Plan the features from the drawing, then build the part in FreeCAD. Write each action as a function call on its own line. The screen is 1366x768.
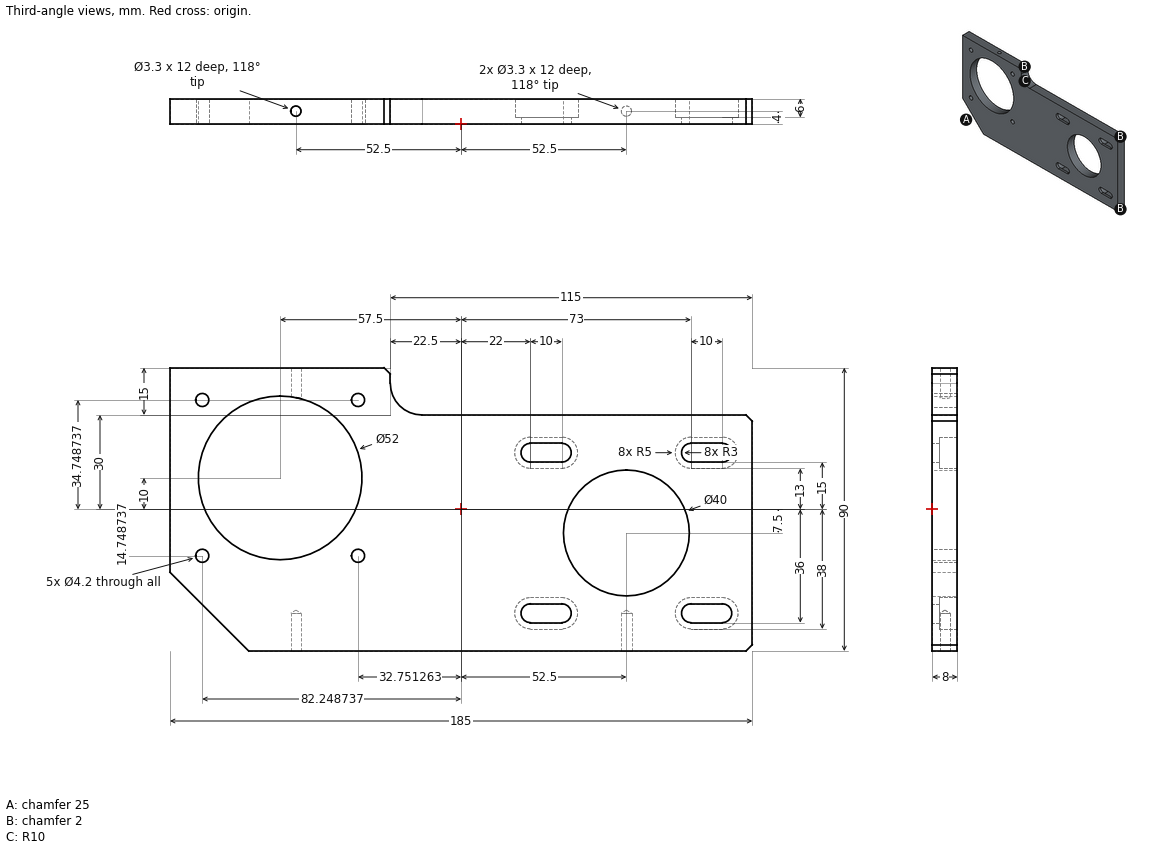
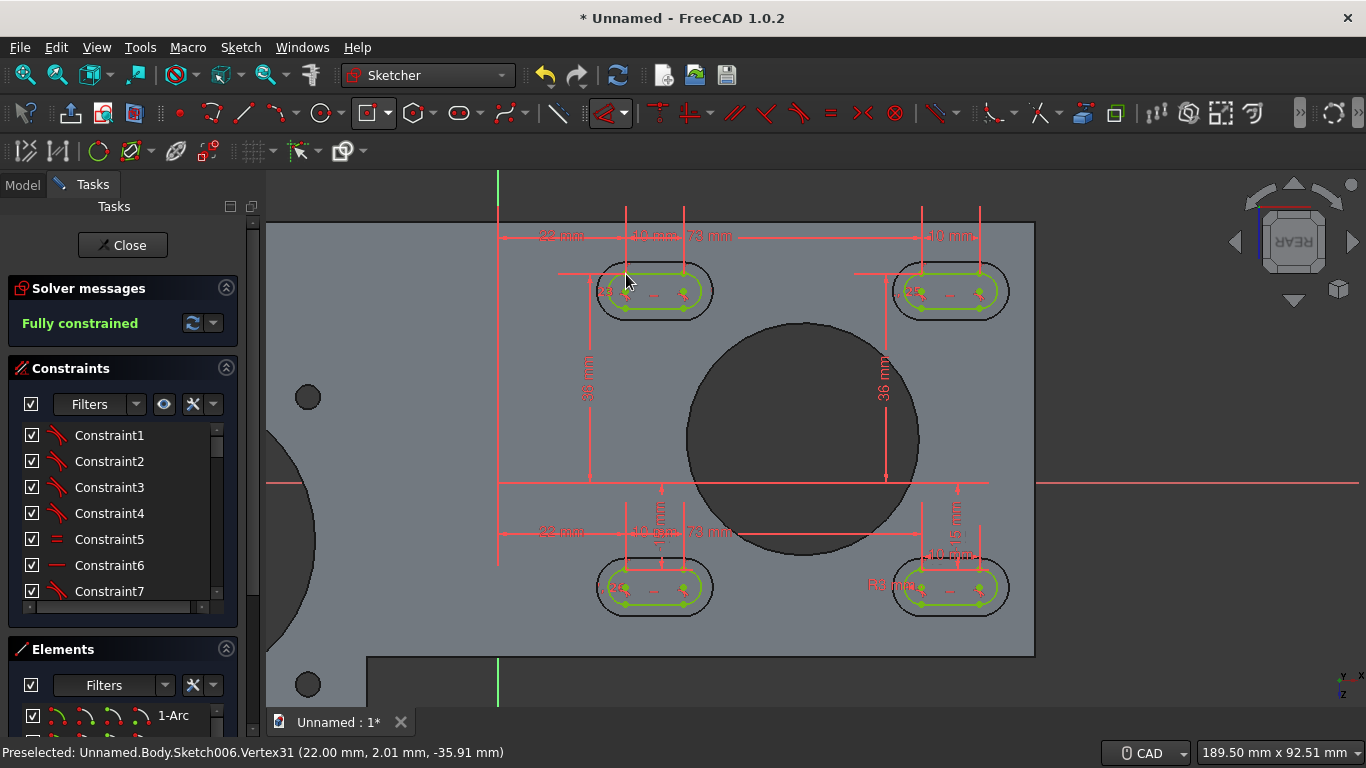
click(123, 245)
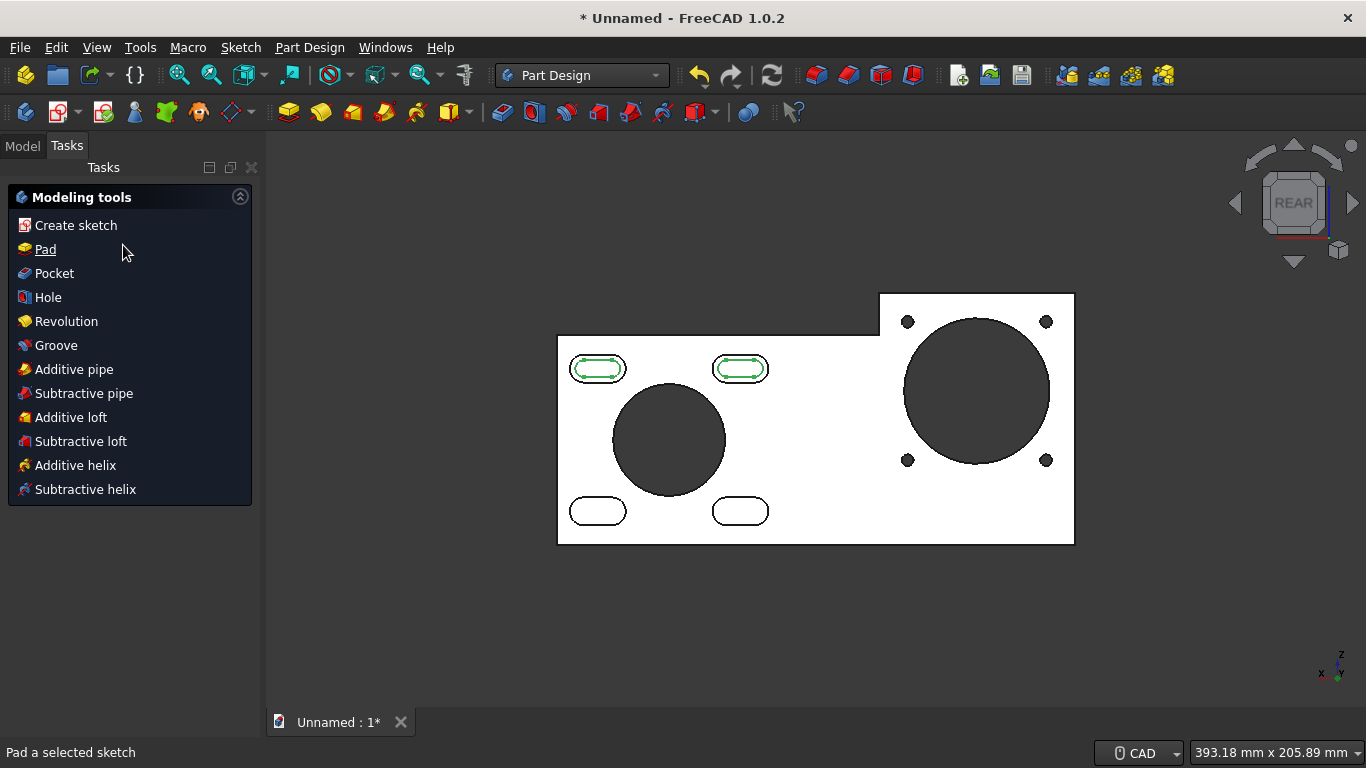
click(504, 112)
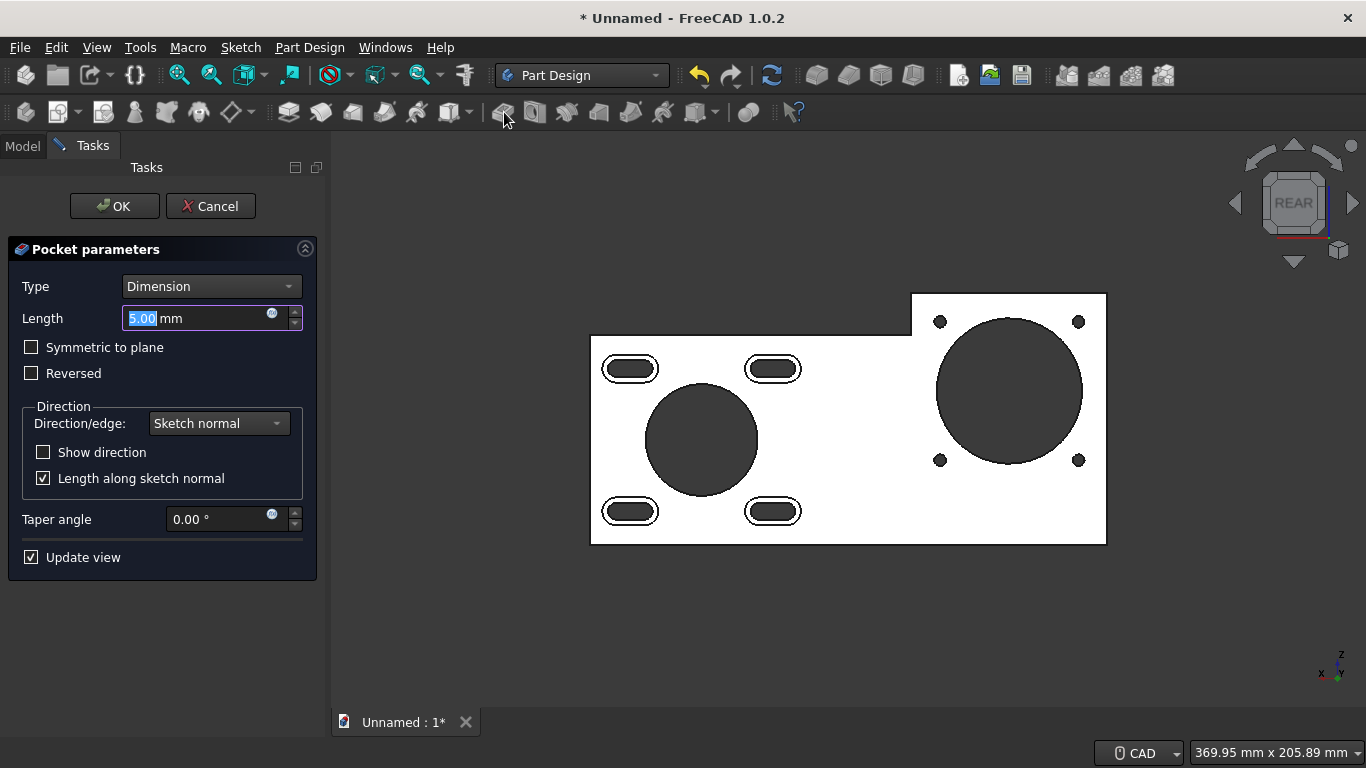
click(212, 286)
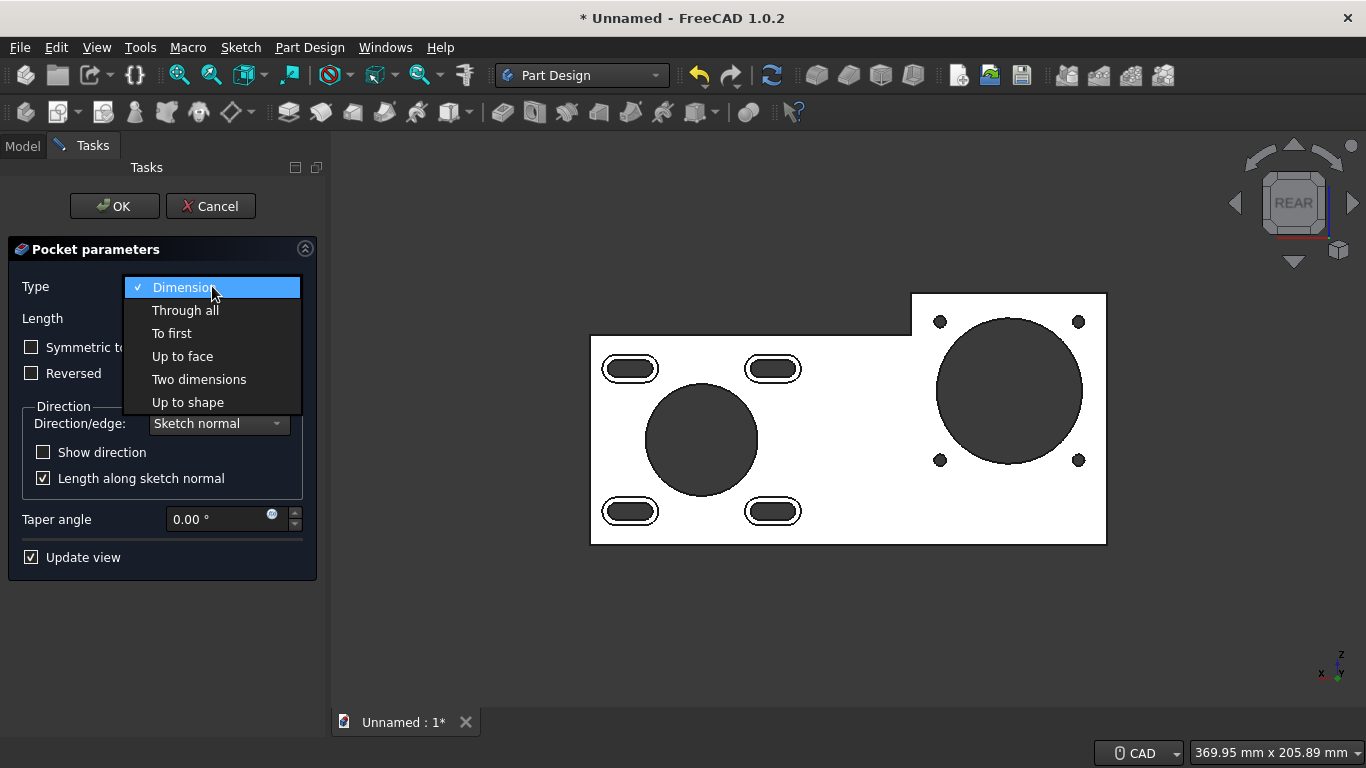
click(212, 310)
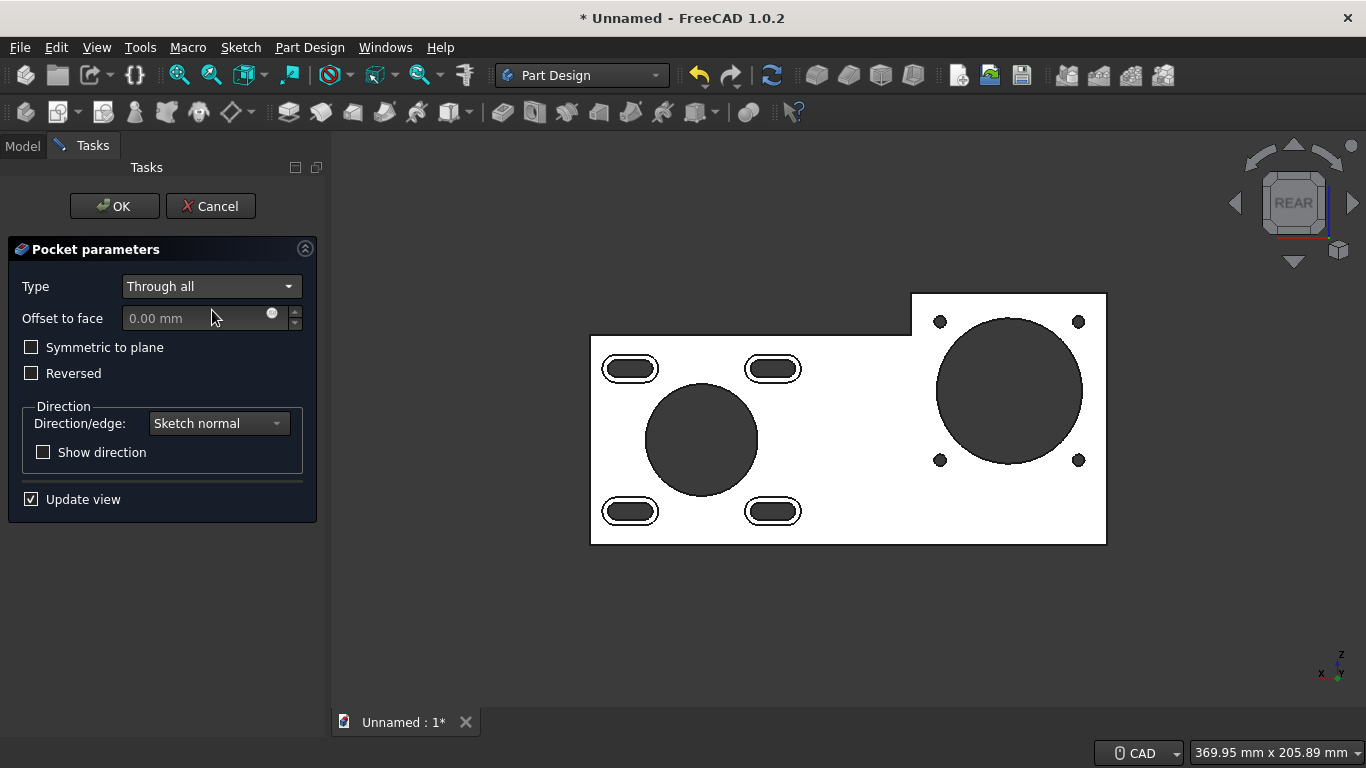
click(115, 206)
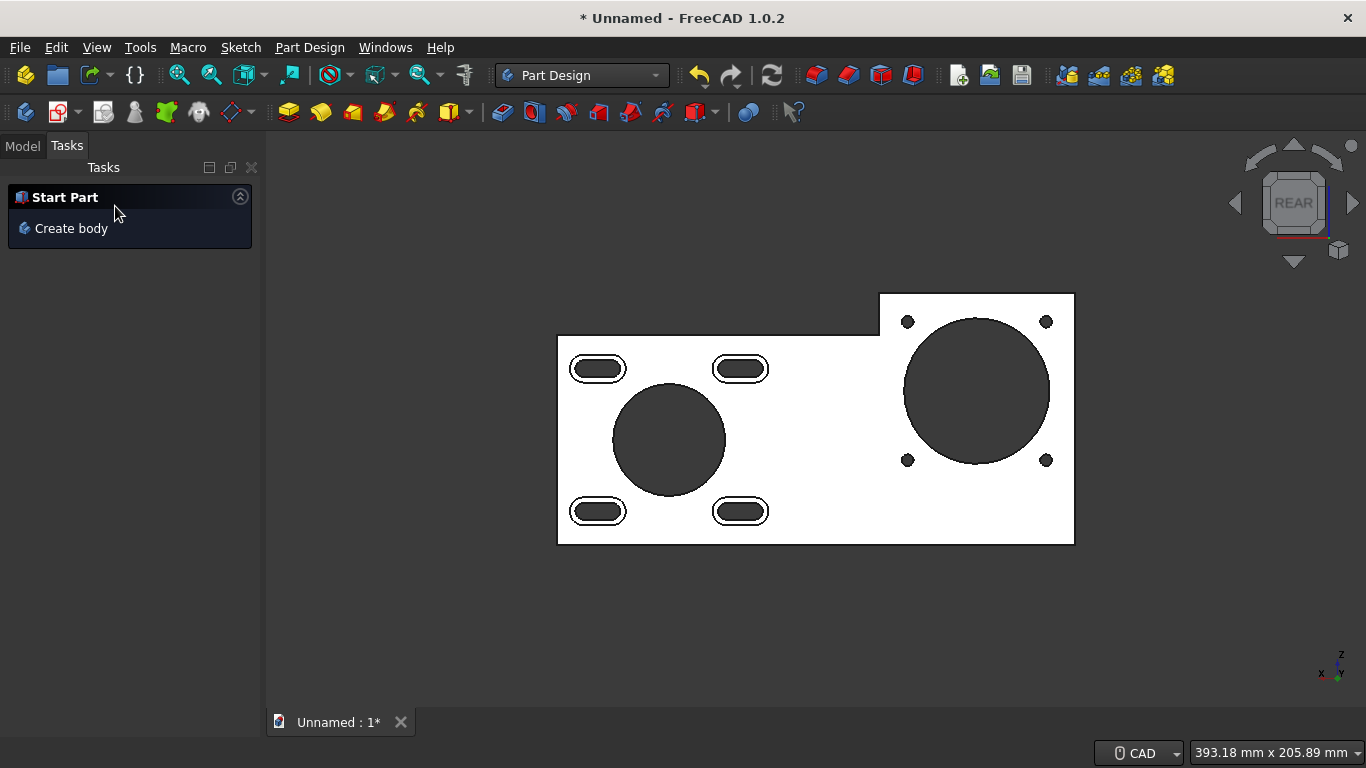
key(5)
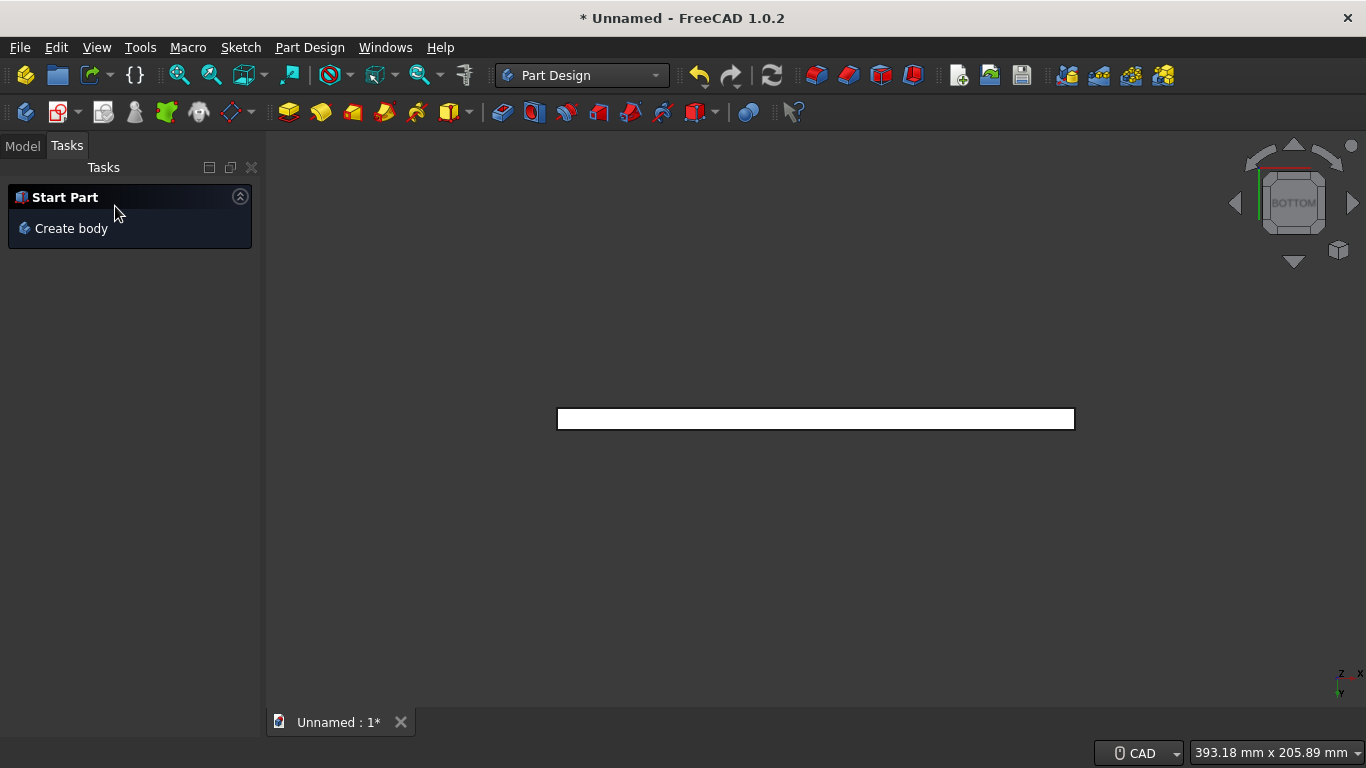
click(1038, 418)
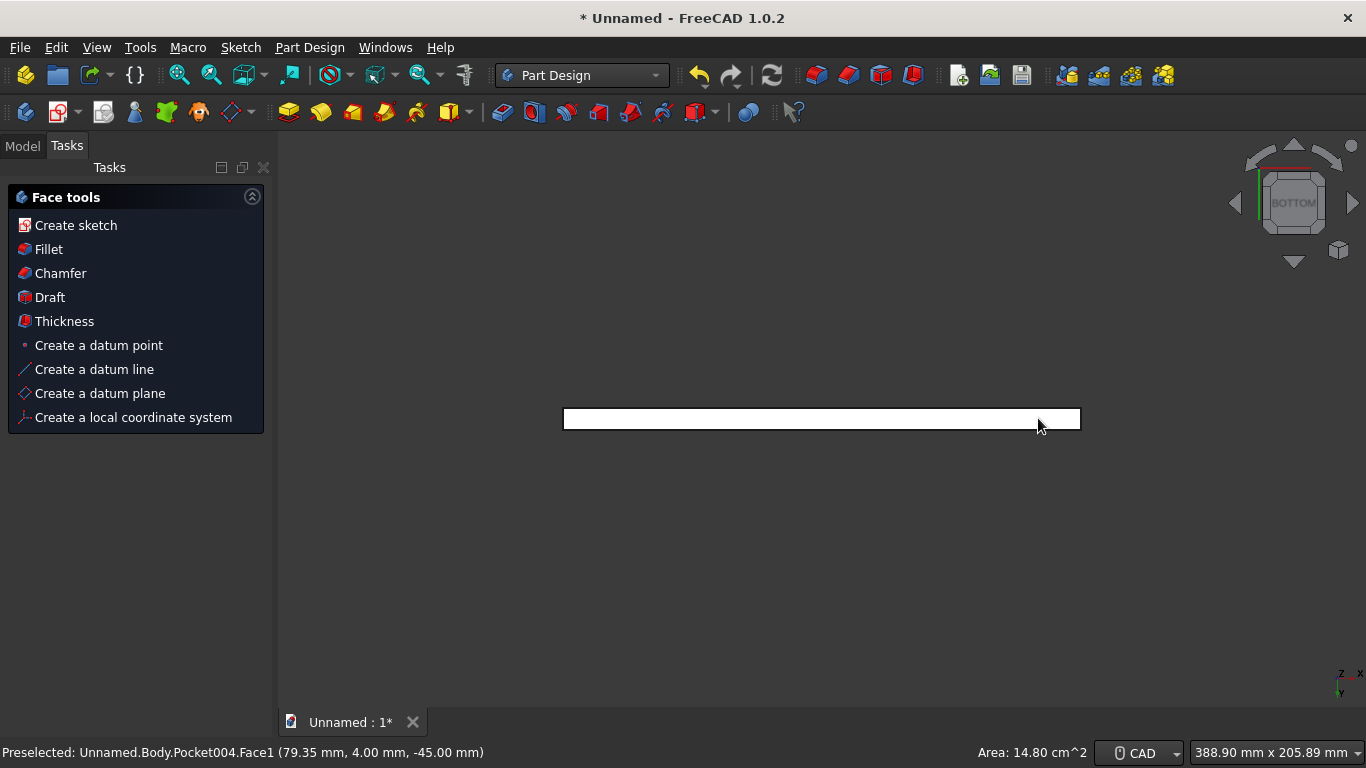
click(58, 112)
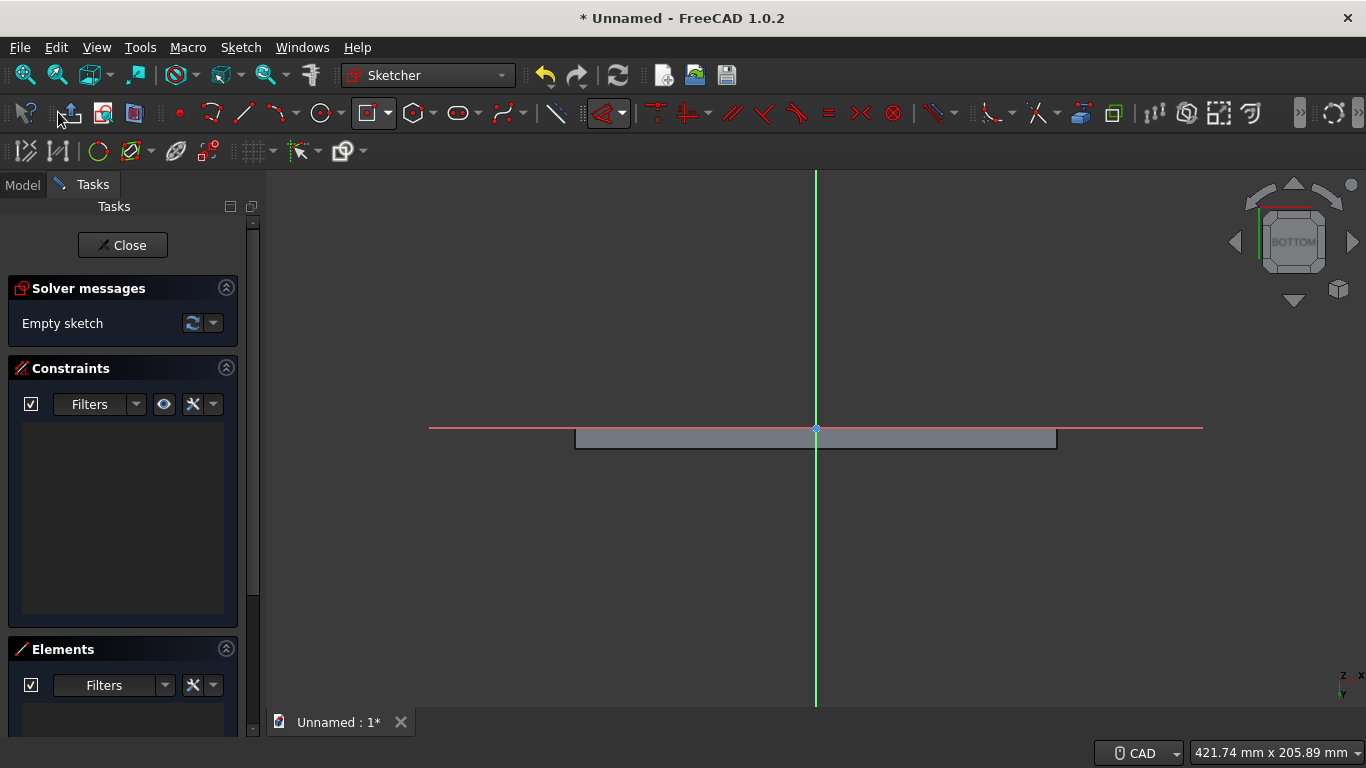
scroll(872, 433, up, 4)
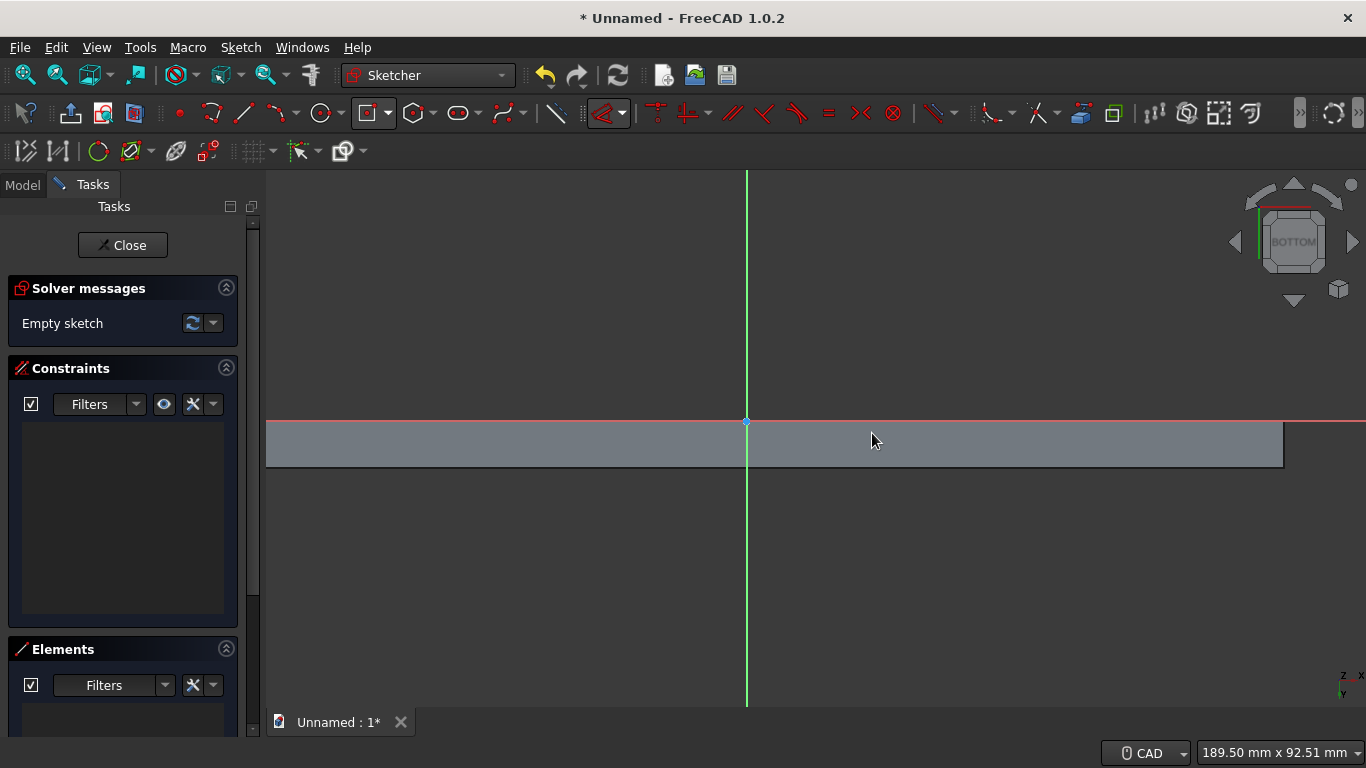
click(322, 114)